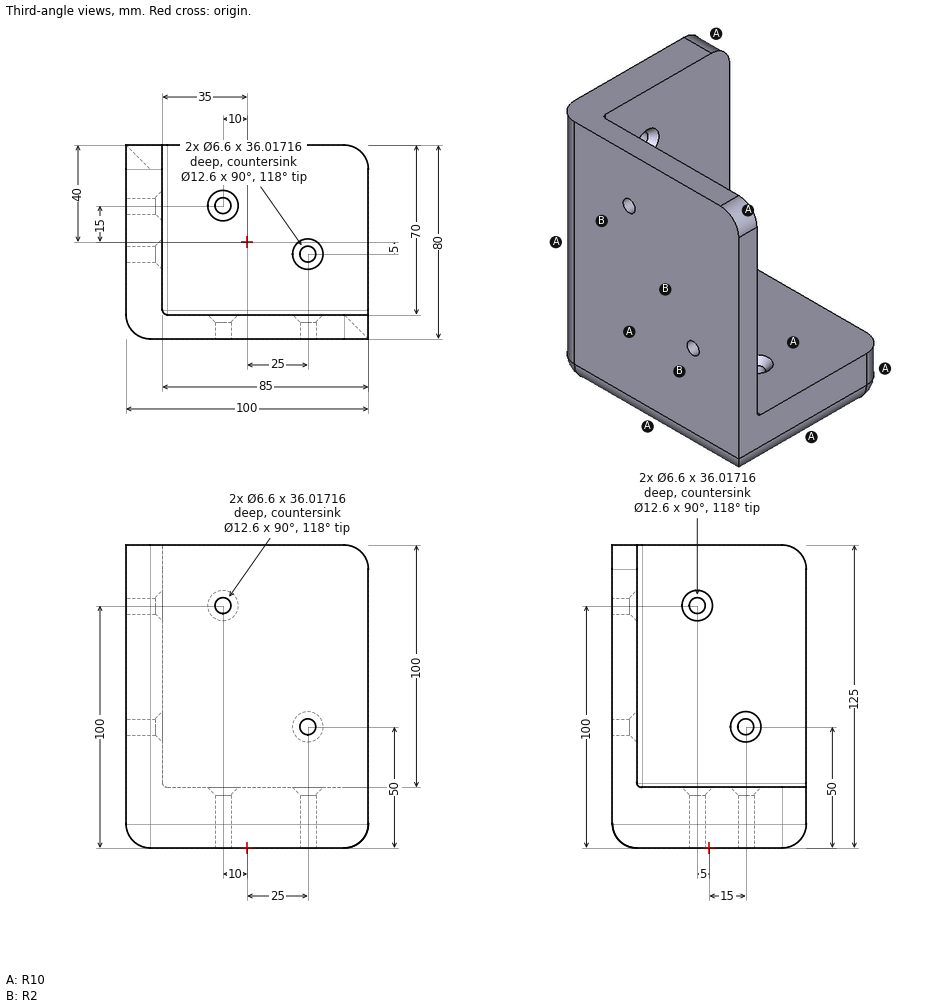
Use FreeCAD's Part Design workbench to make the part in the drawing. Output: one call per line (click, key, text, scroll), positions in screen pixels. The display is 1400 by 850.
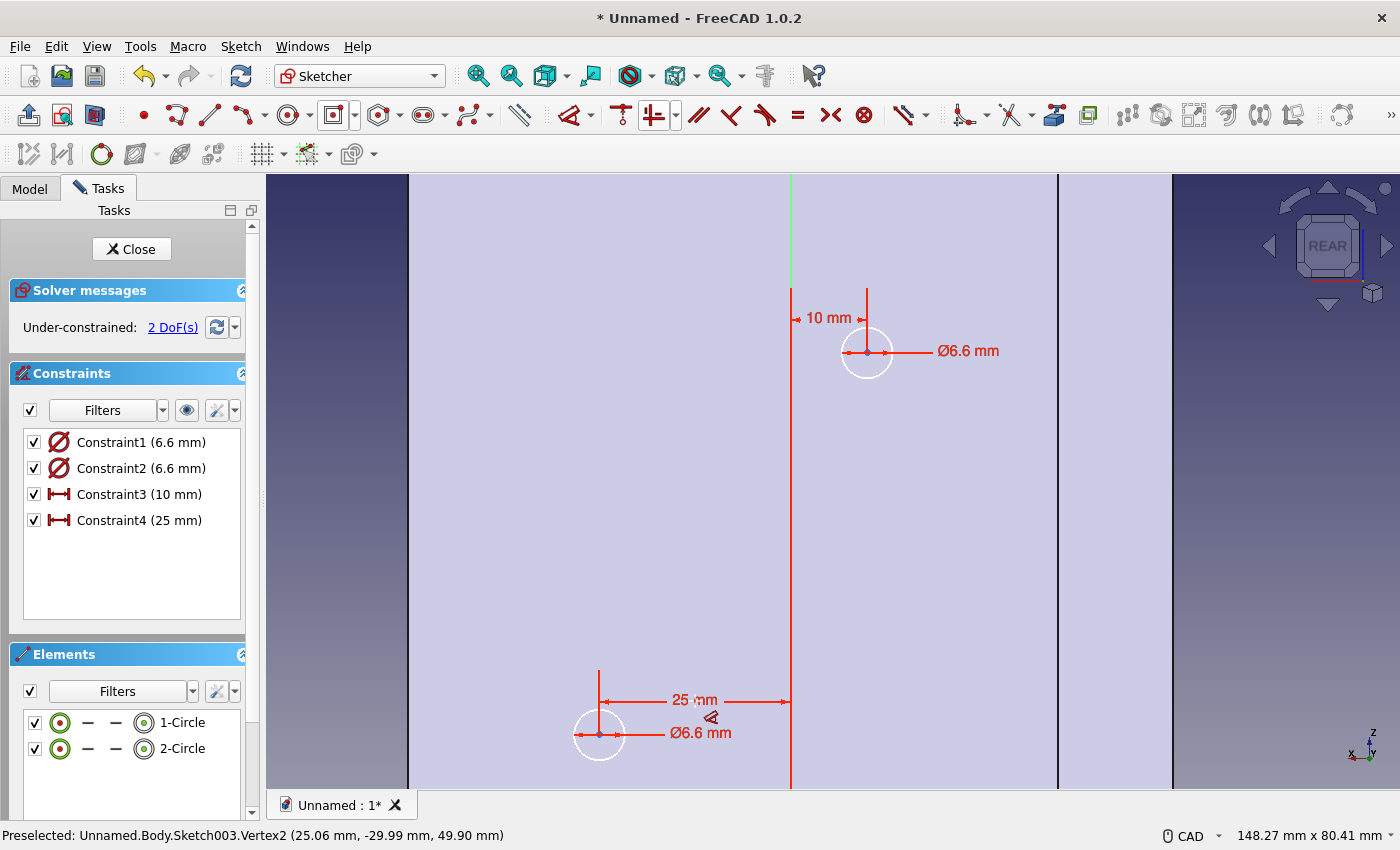
click(599, 735)
click(565, 754)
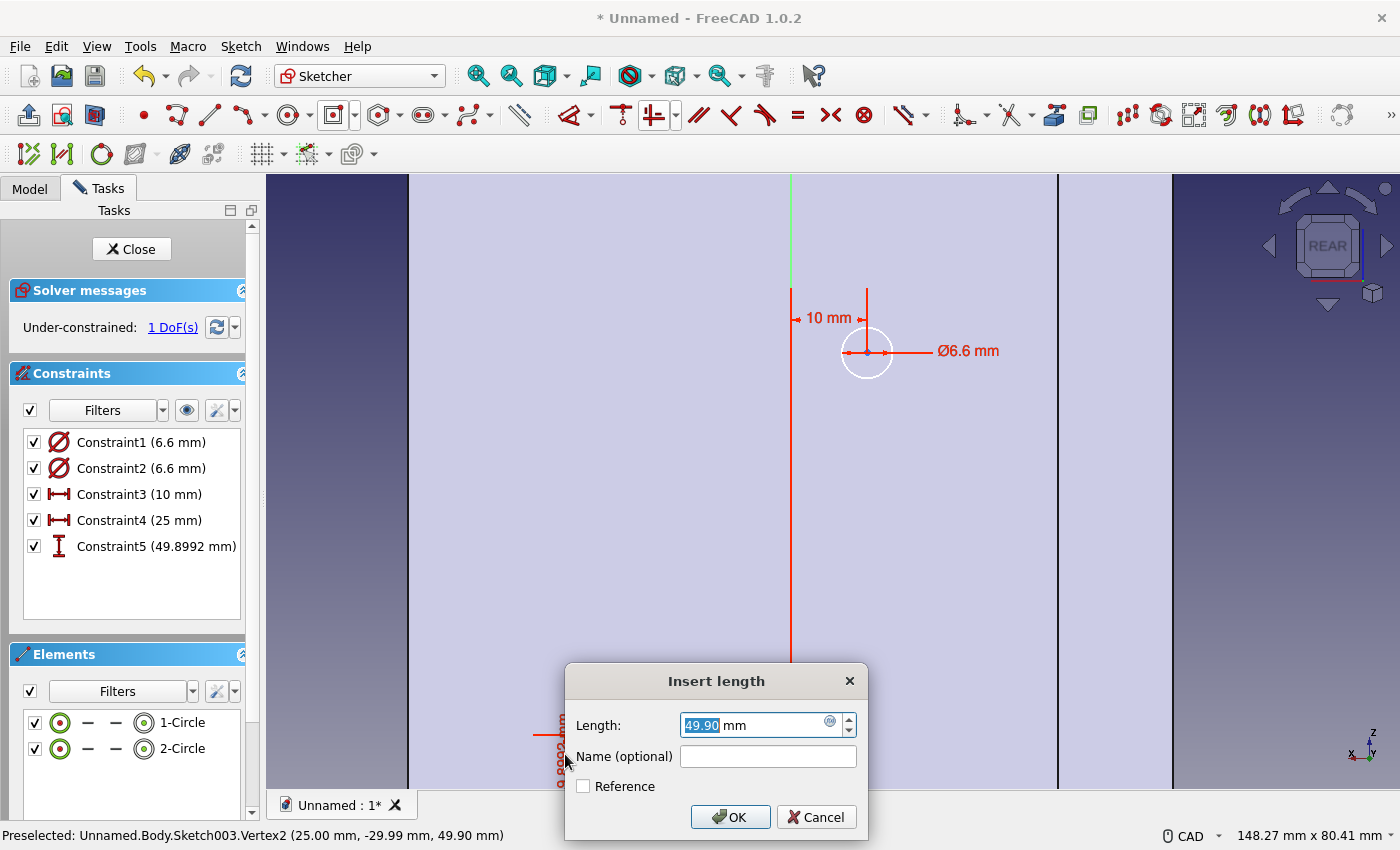
text(50)
key(Return)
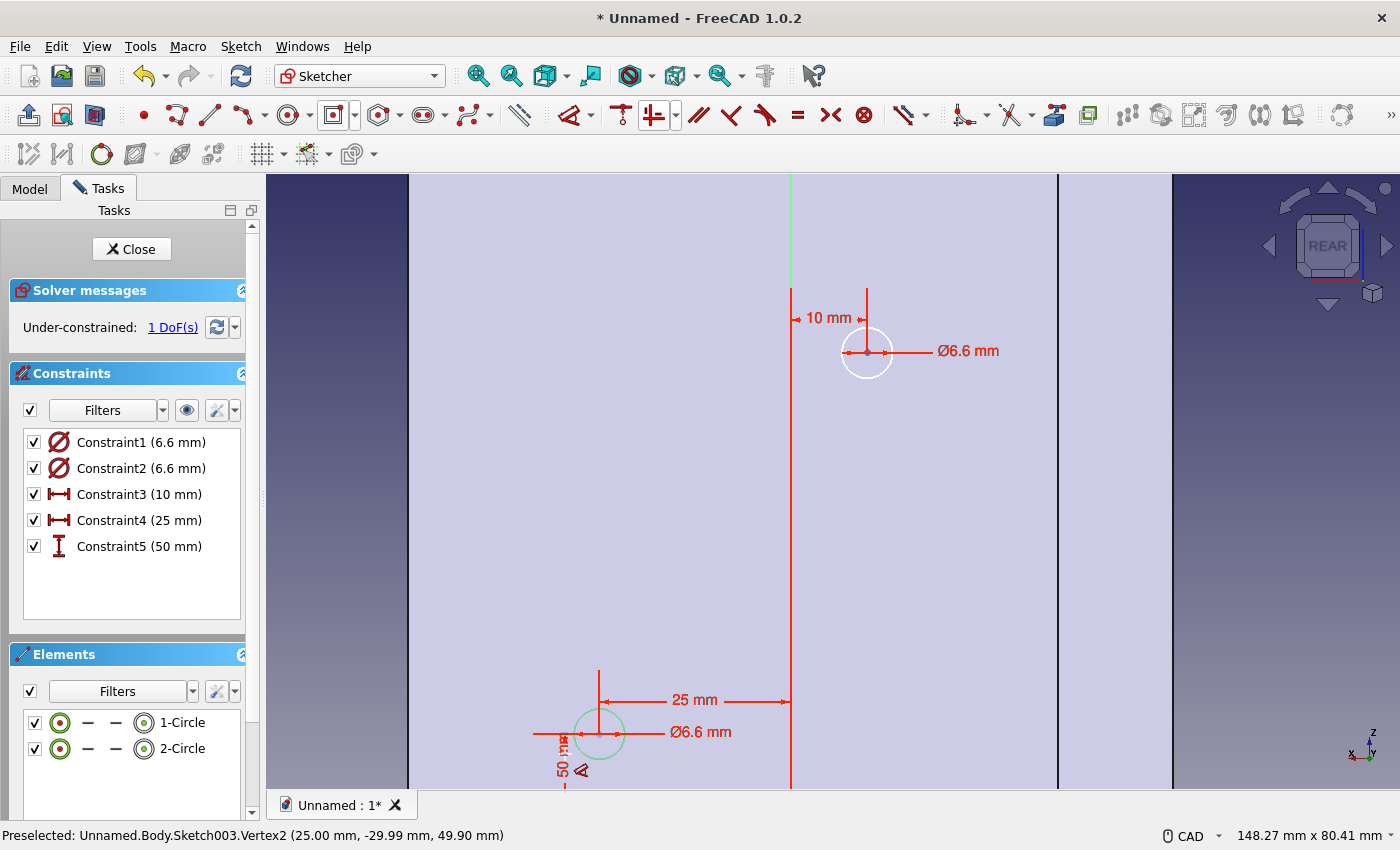
click(867, 353)
click(901, 557)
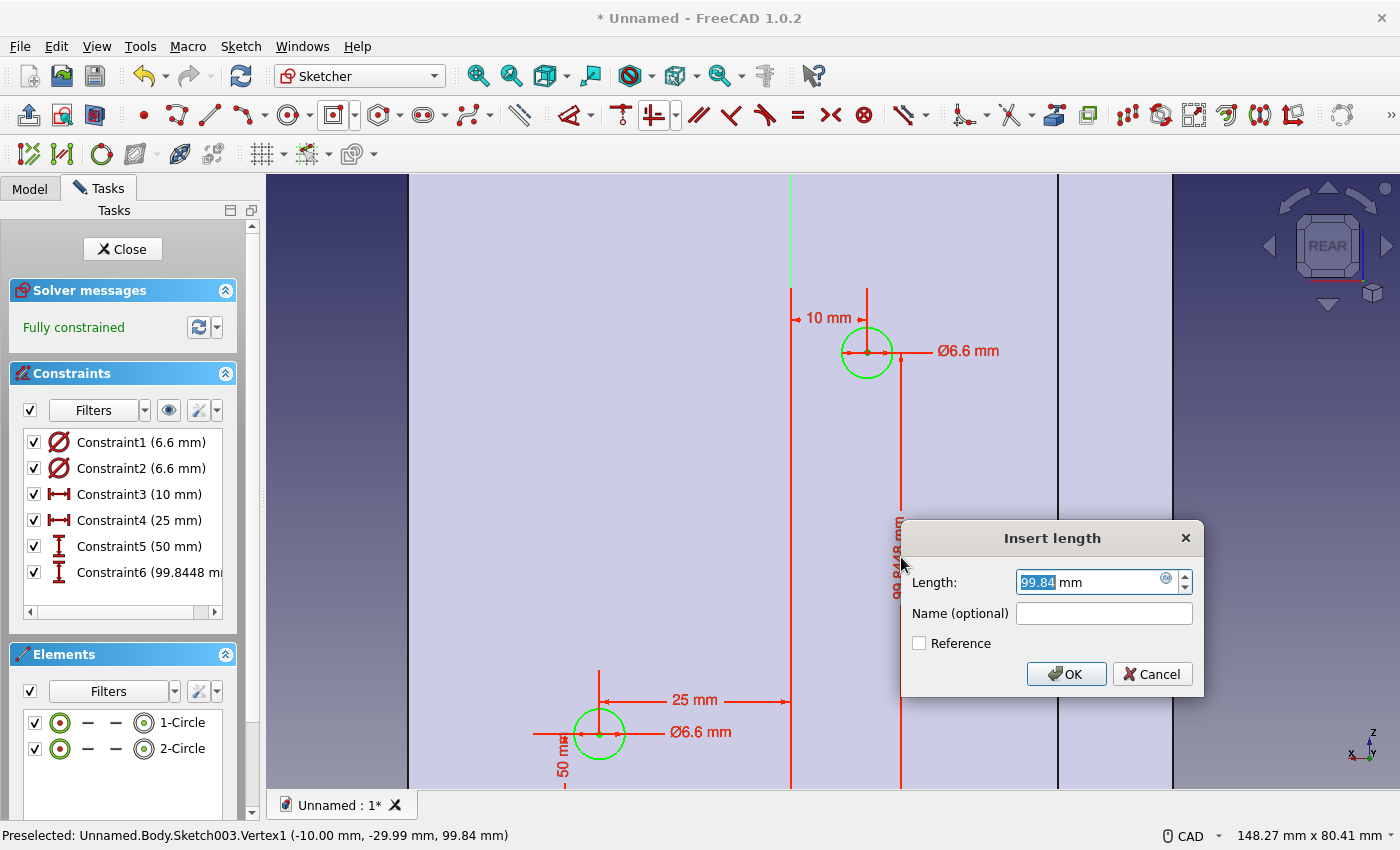
text(100)
key(Return)
key(Escape)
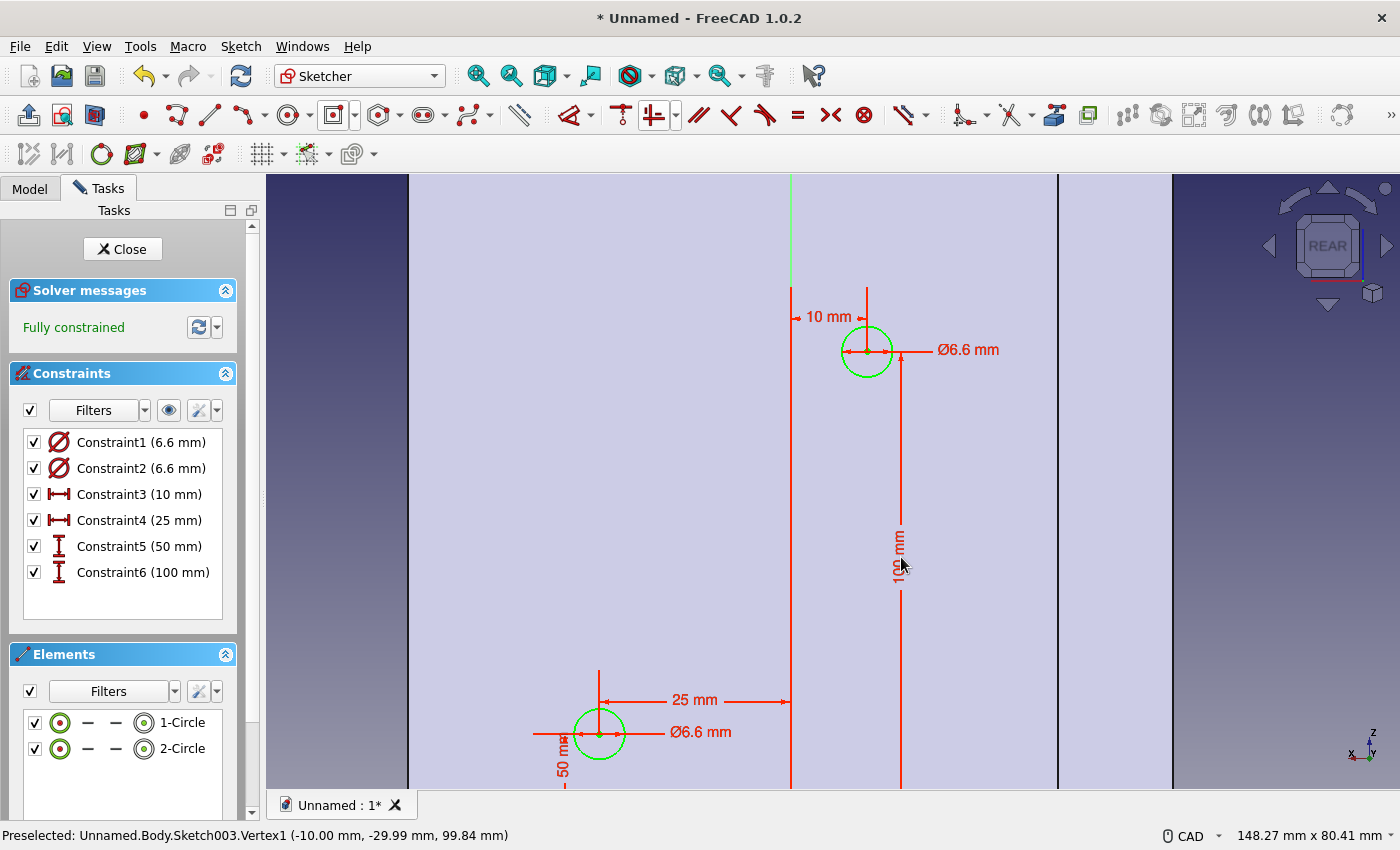
click(123, 249)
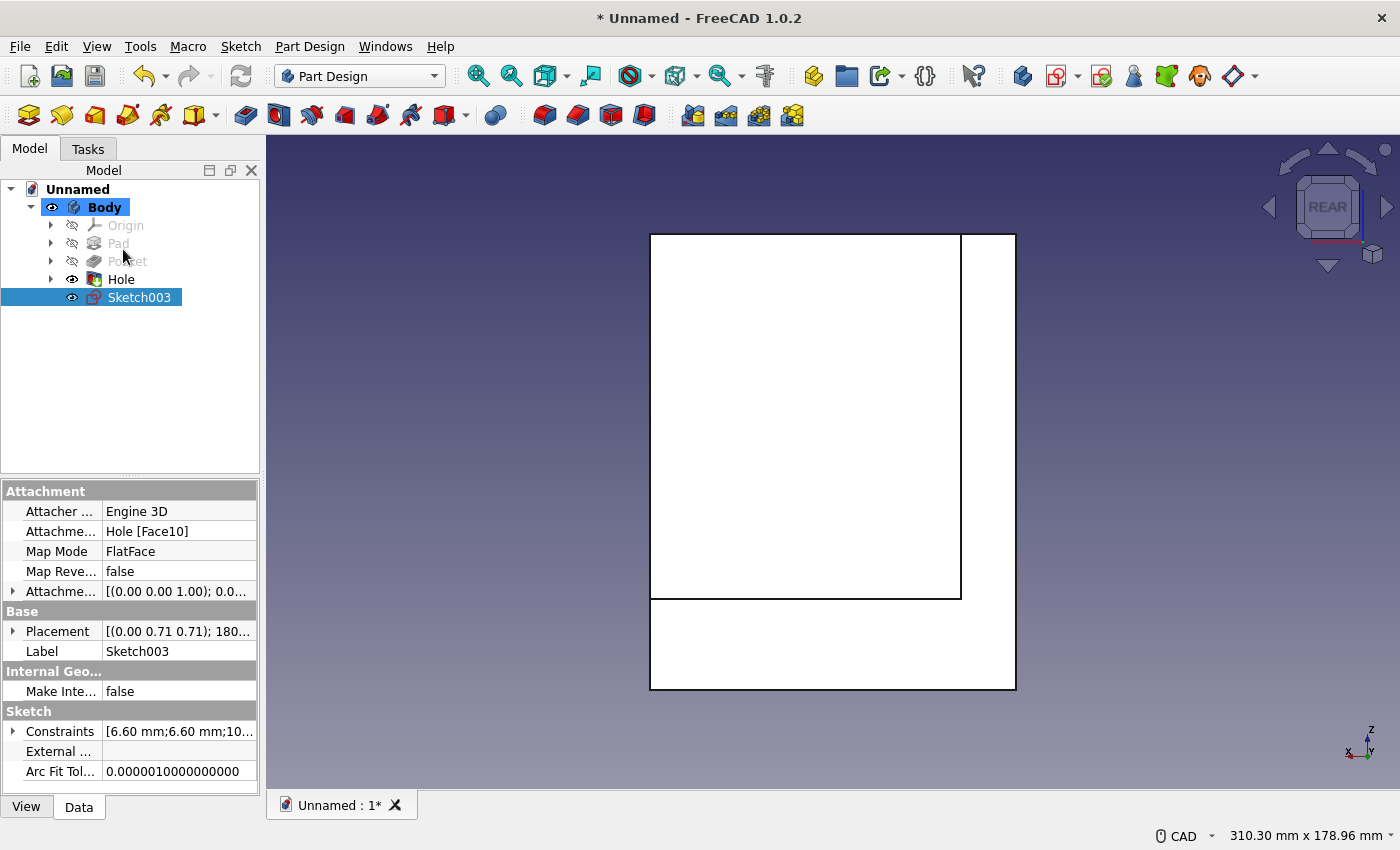
click(279, 116)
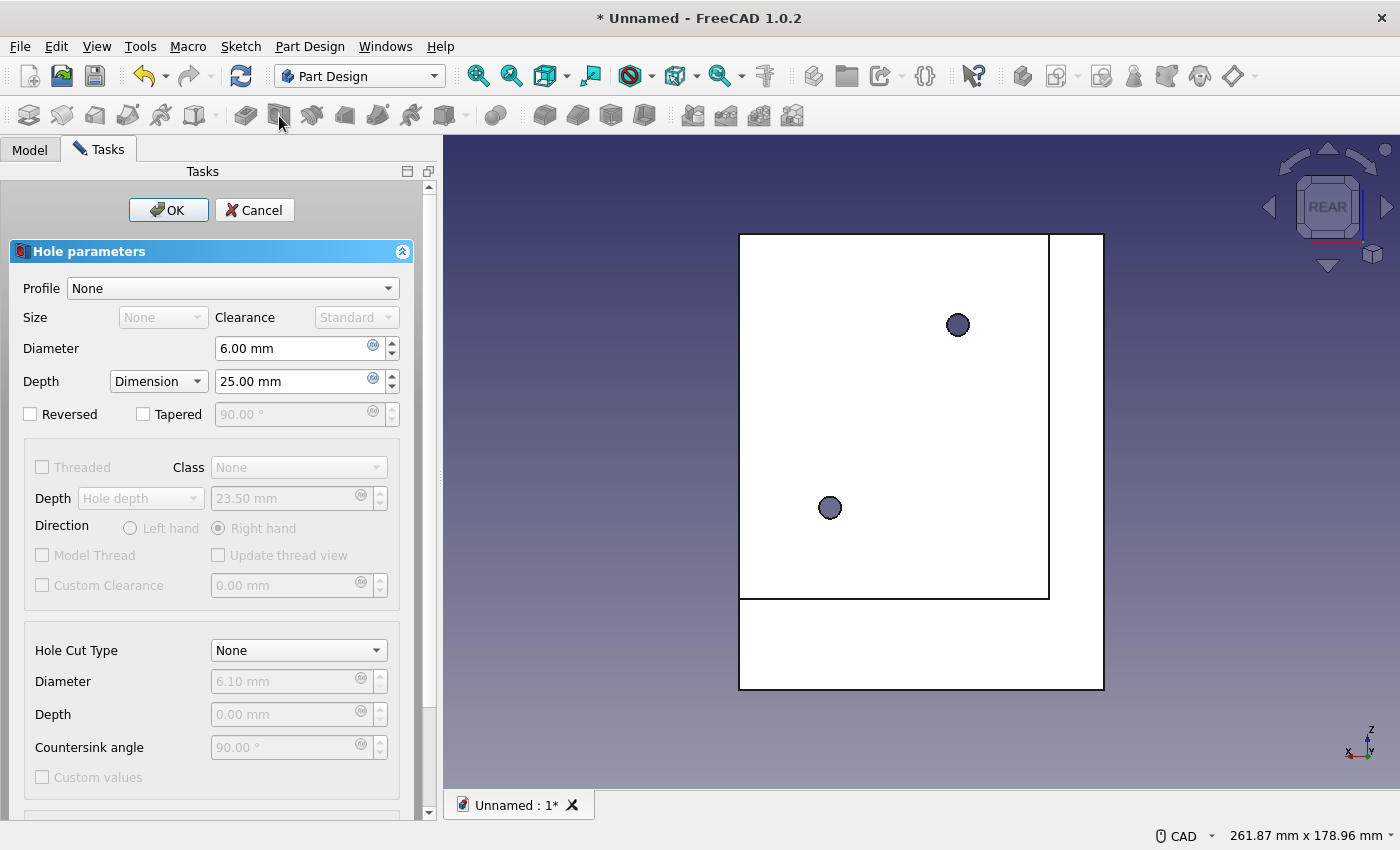
triple_click(300, 348)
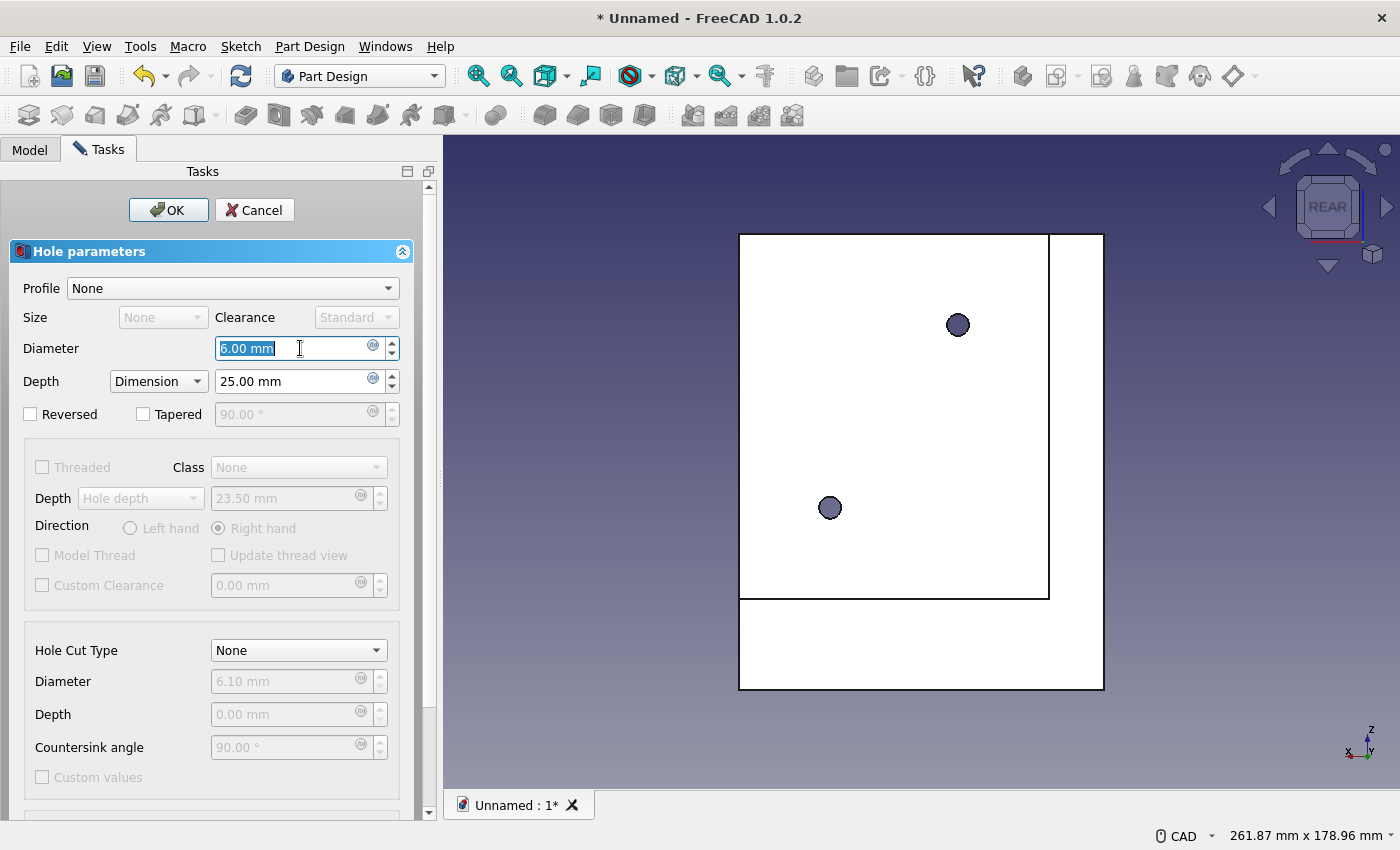
text(6.6)
key(Tab)